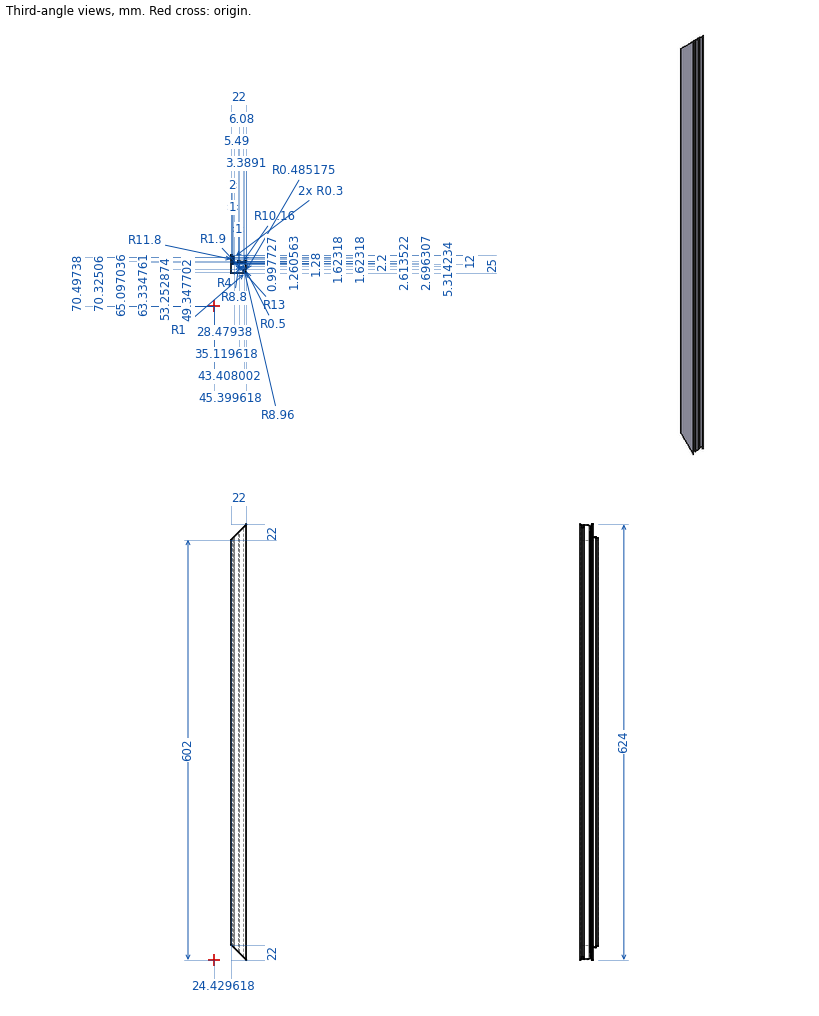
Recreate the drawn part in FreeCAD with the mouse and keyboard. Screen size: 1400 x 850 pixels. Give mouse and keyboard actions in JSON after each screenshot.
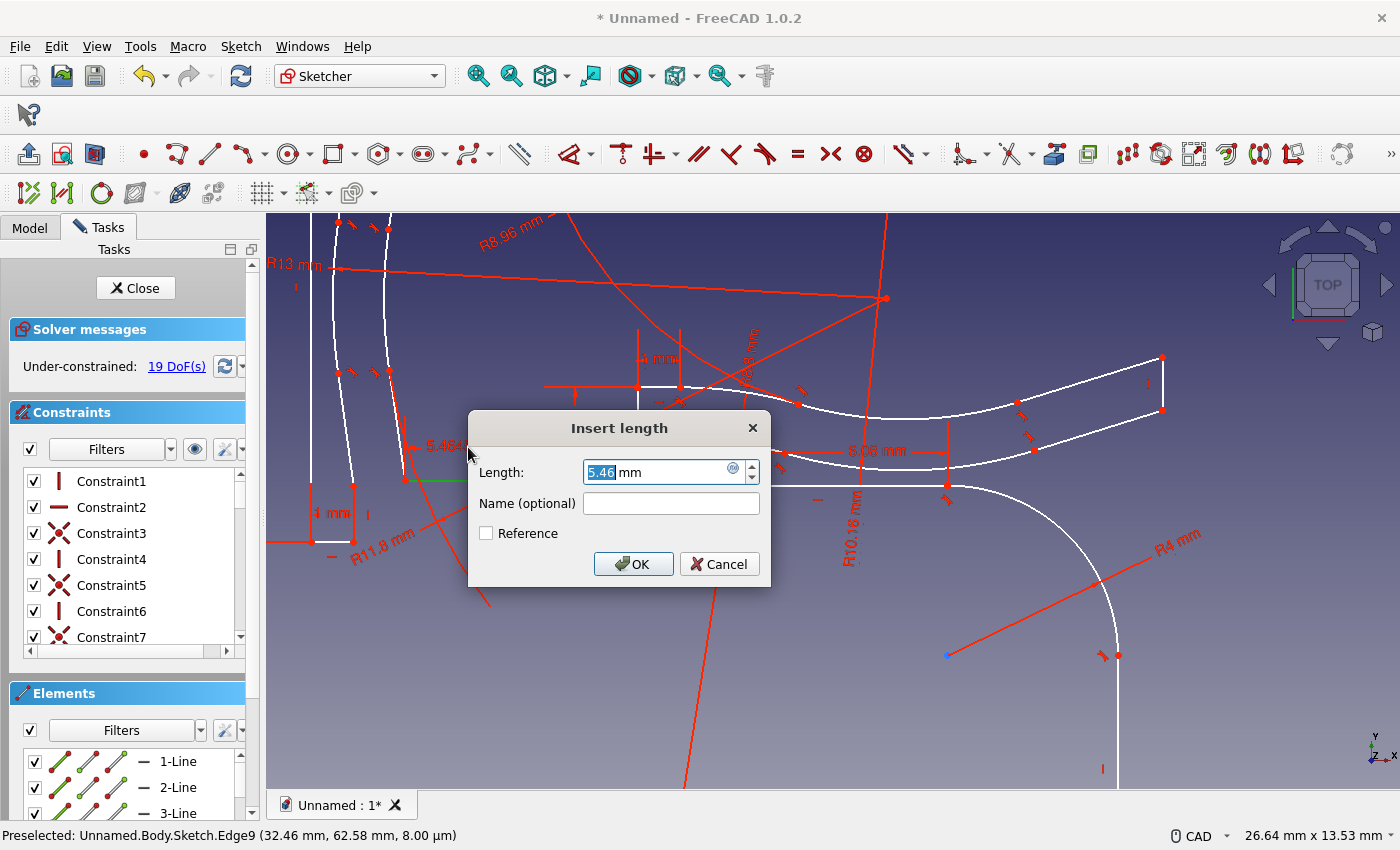
{"action": "type", "text": "5.49"}
{"action": "key", "text": "Return"}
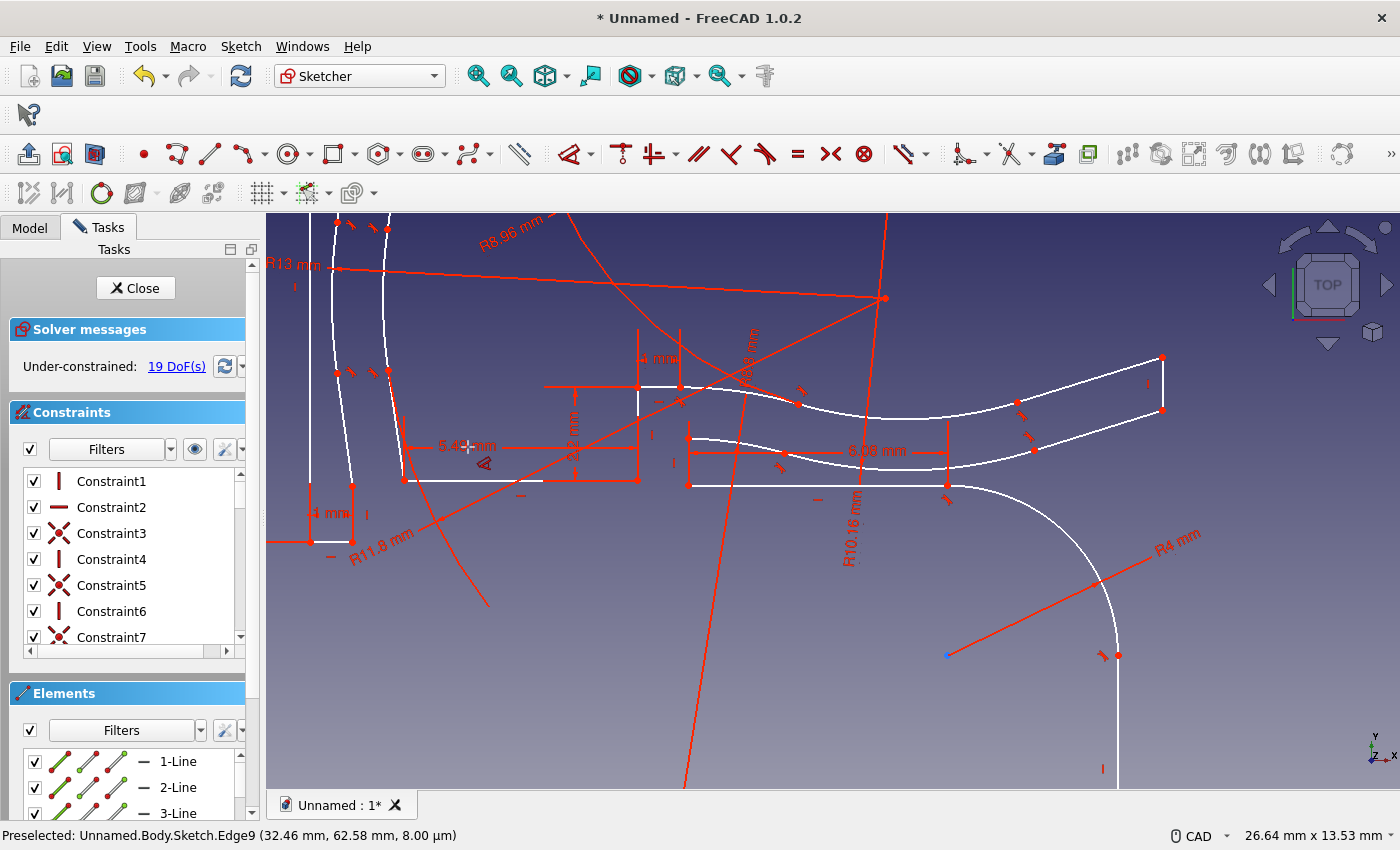
{"action": "left_click", "coordinate": [353, 503]}
{"action": "left_click", "coordinate": [387, 534]}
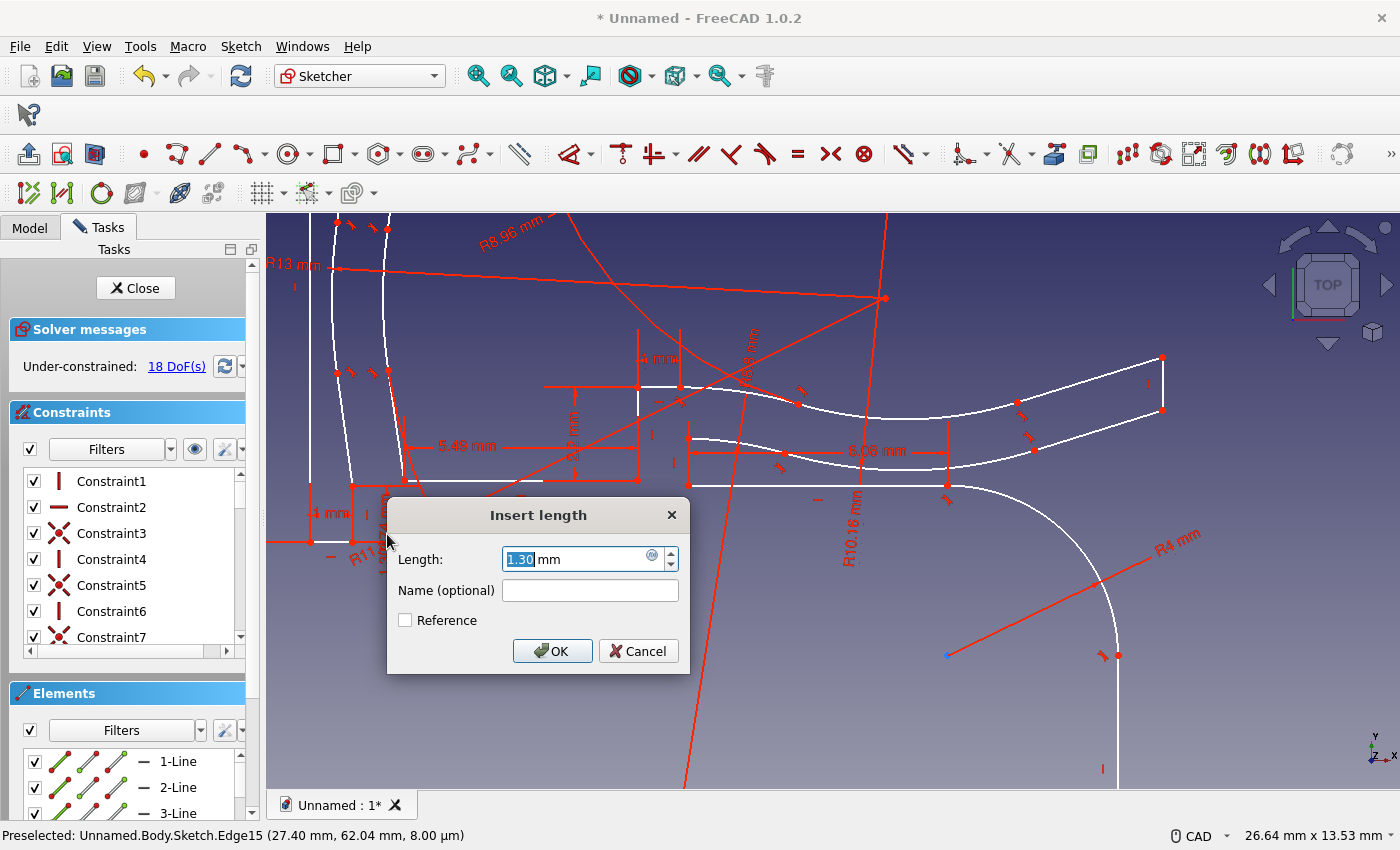
{"action": "type", "text": "1.28"}
{"action": "key", "text": "Return"}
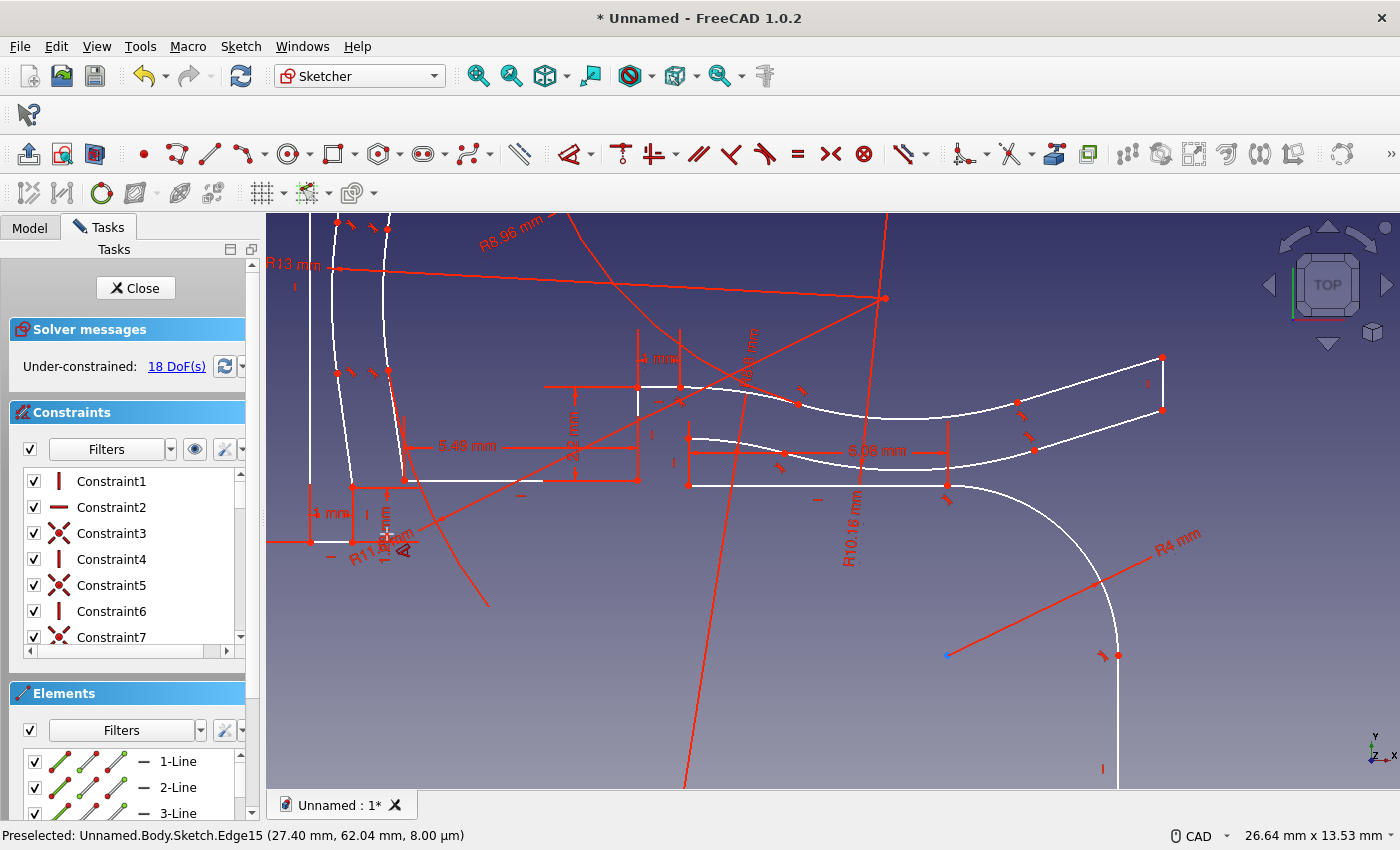
{"action": "left_click", "coordinate": [1119, 371]}
{"action": "left_click", "coordinate": [1090, 323]}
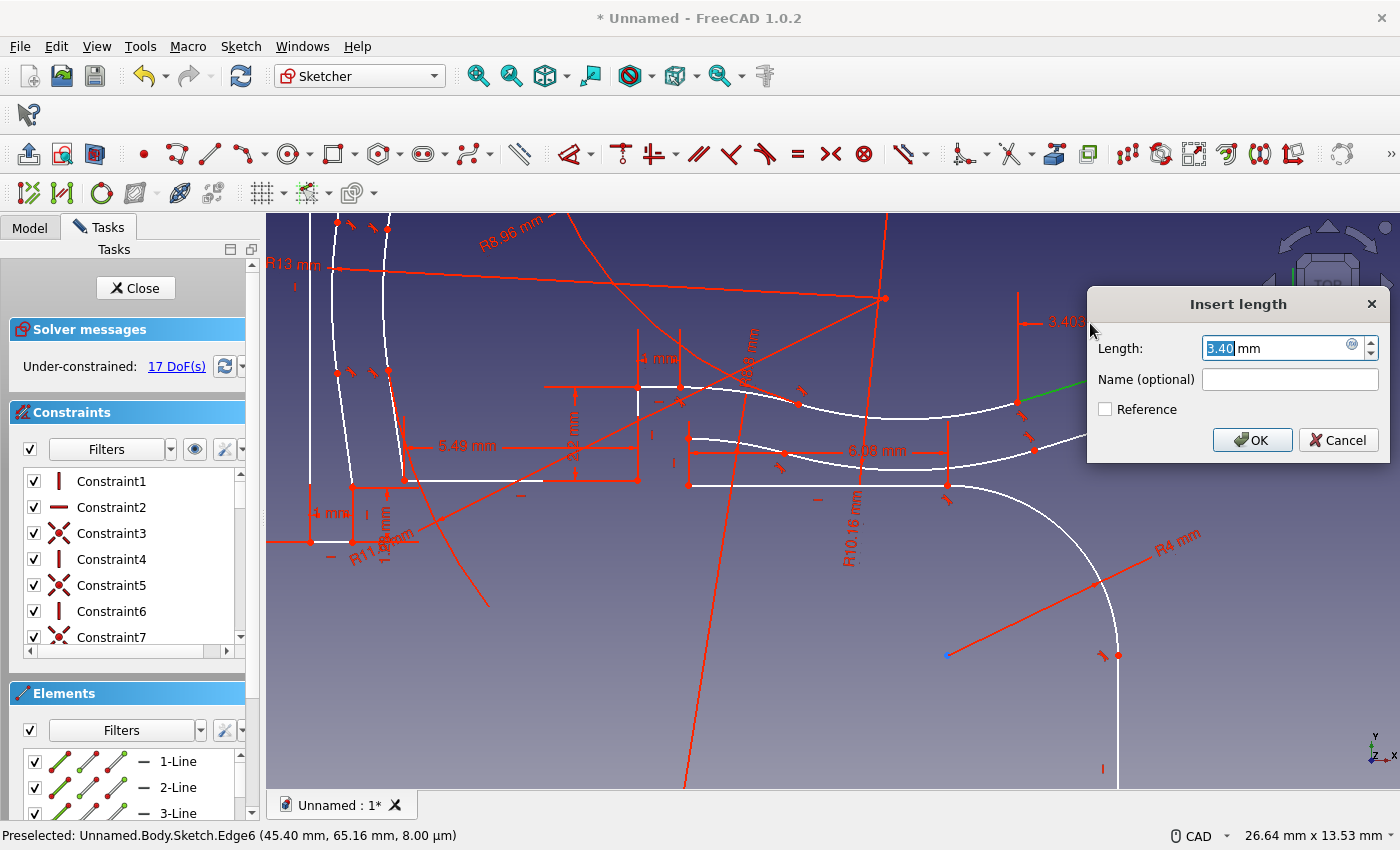
{"action": "type", "text": "3.3891"}
{"action": "key", "text": "Return"}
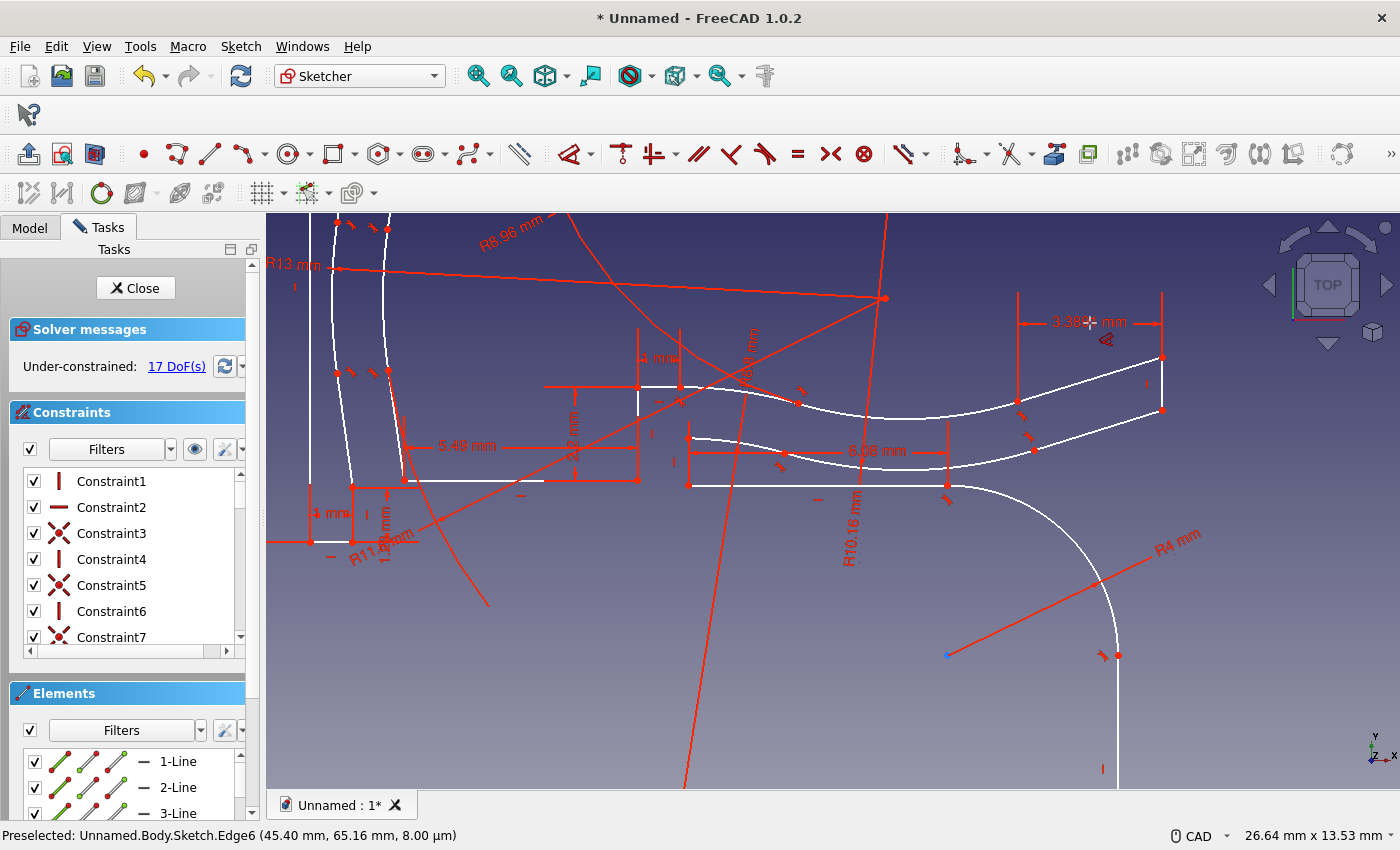
{"action": "left_click", "coordinate": [1118, 723]}
{"action": "left_click", "coordinate": [1152, 708]}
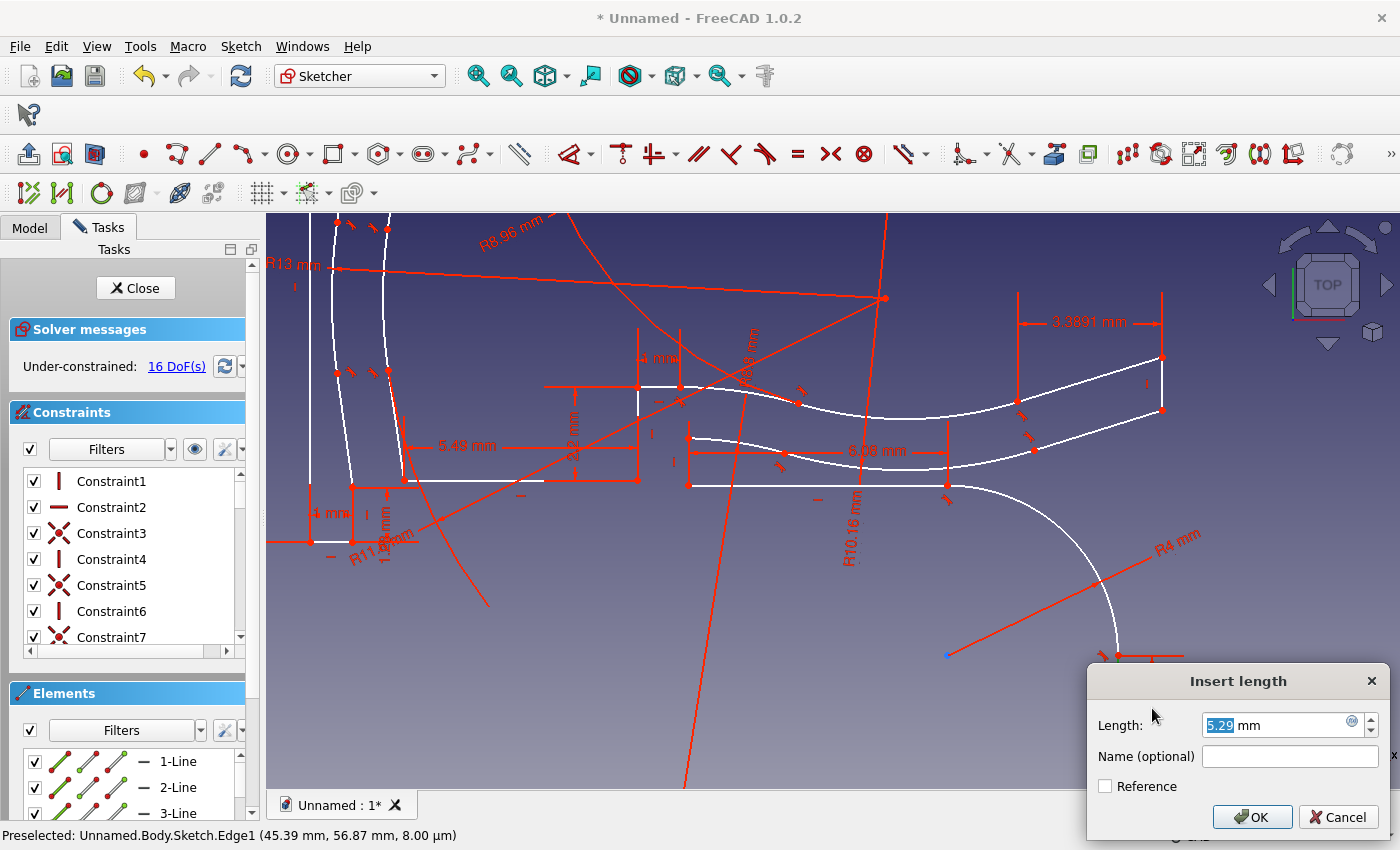
{"action": "type", "text": "5.314234"}
{"action": "key", "text": "Return"}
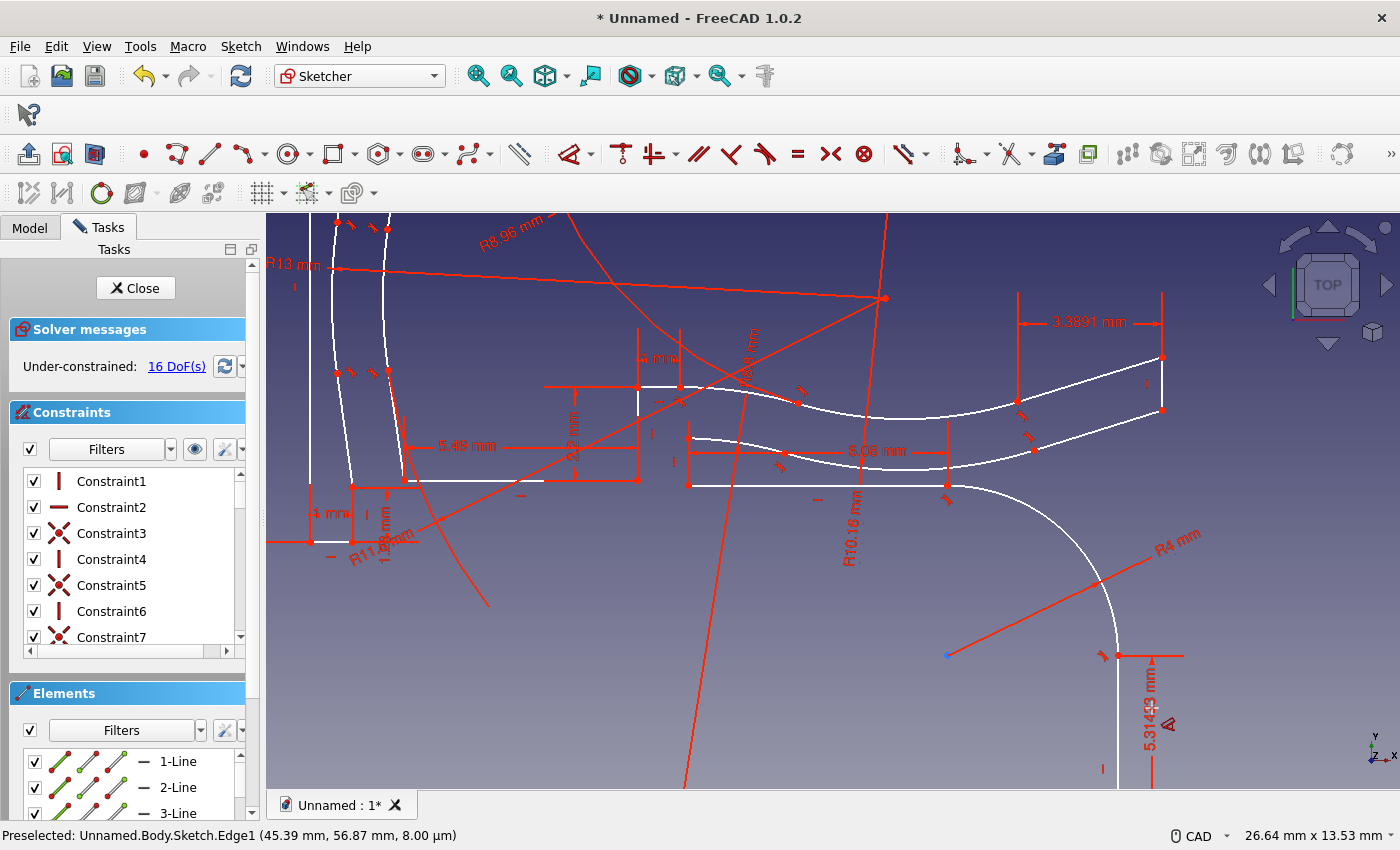
{"action": "left_click", "coordinate": [689, 471]}
{"action": "left_click", "coordinate": [655, 462]}